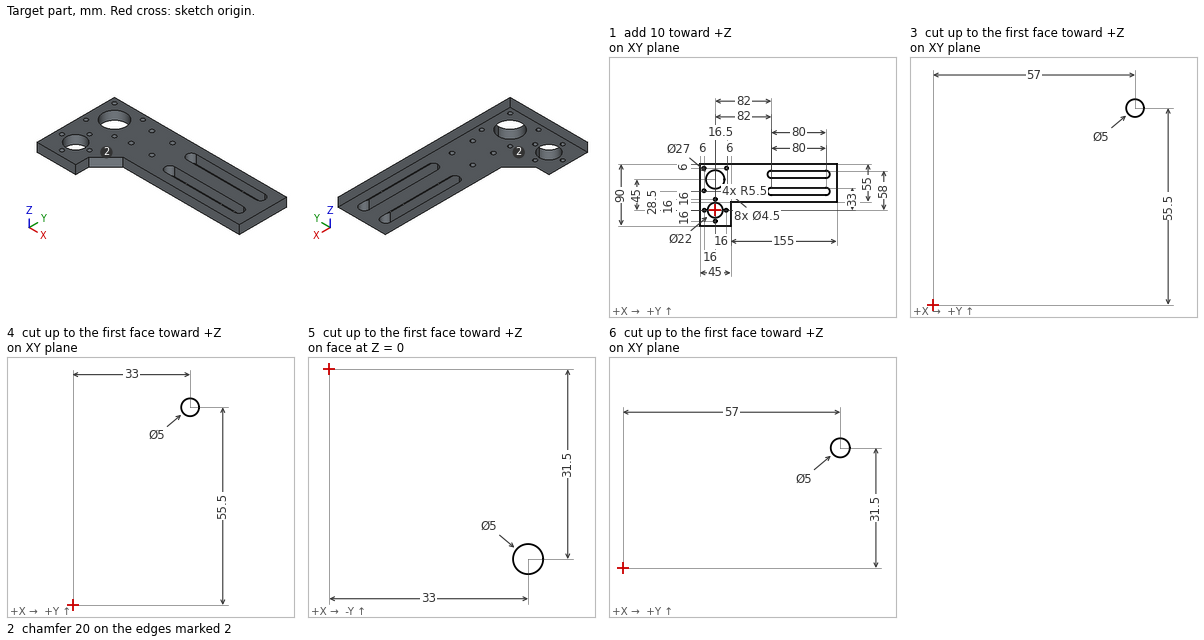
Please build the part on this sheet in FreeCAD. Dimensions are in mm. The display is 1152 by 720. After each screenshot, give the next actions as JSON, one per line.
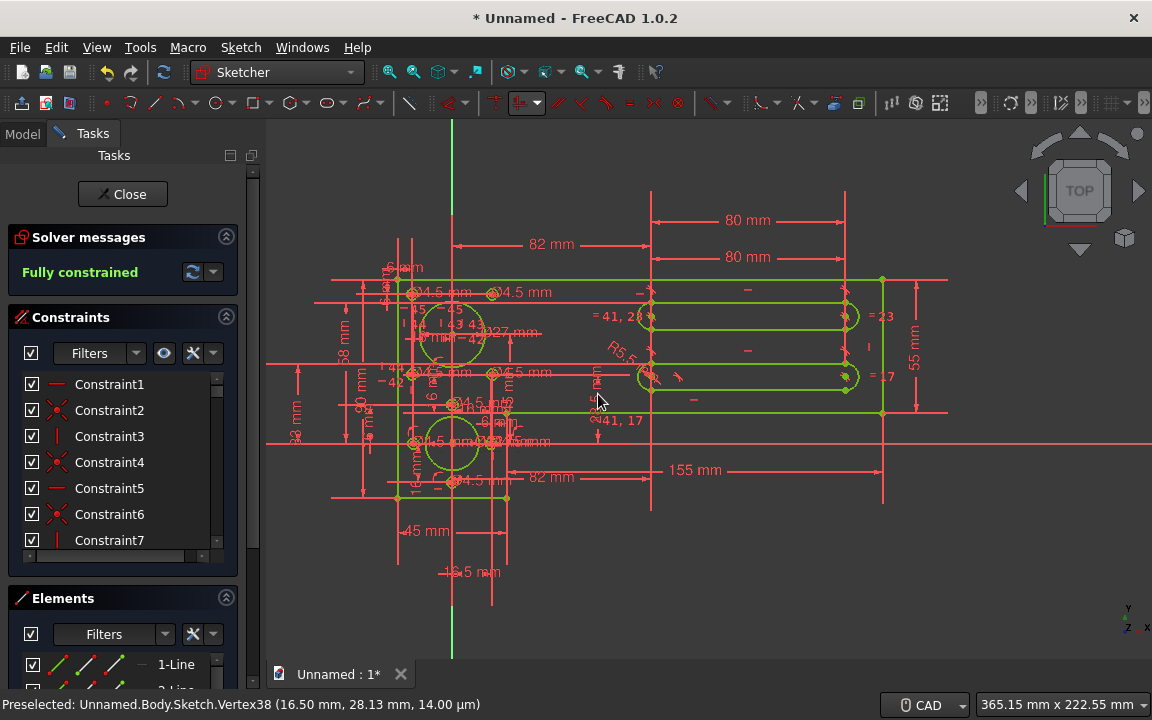
{"action": "left_click", "coordinate": [123, 194]}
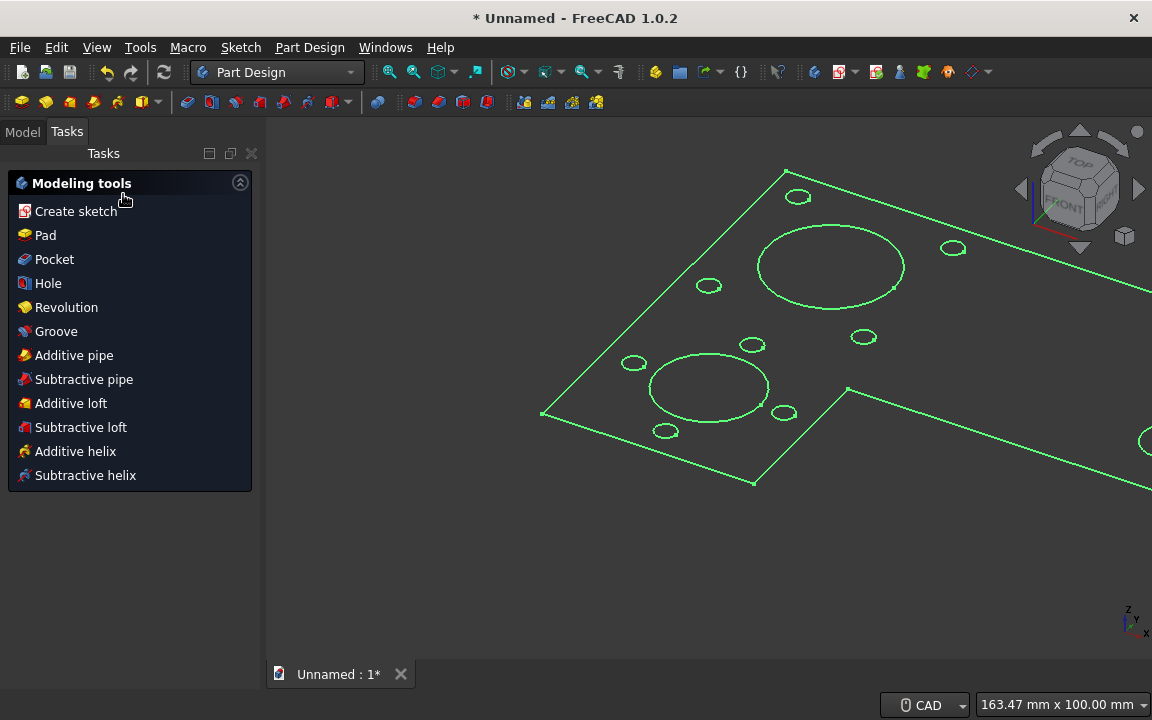
{"action": "left_click", "coordinate": [22, 102]}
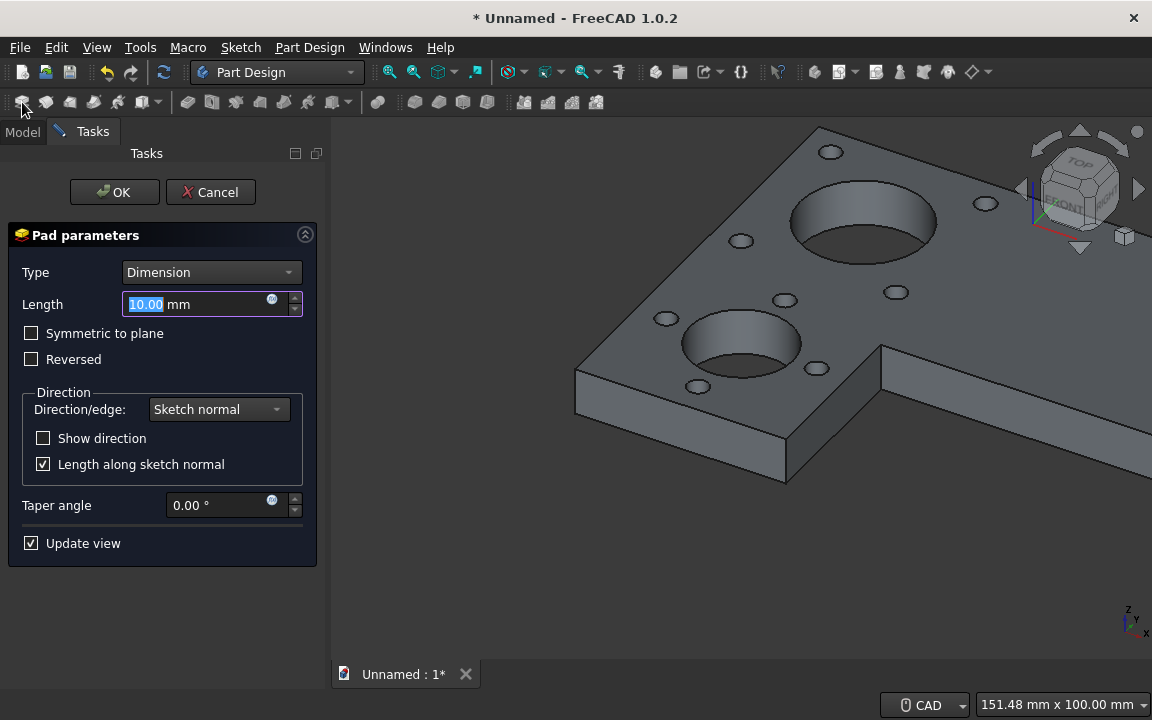
{"action": "type", "text": "10"}
{"action": "key", "text": "Tab"}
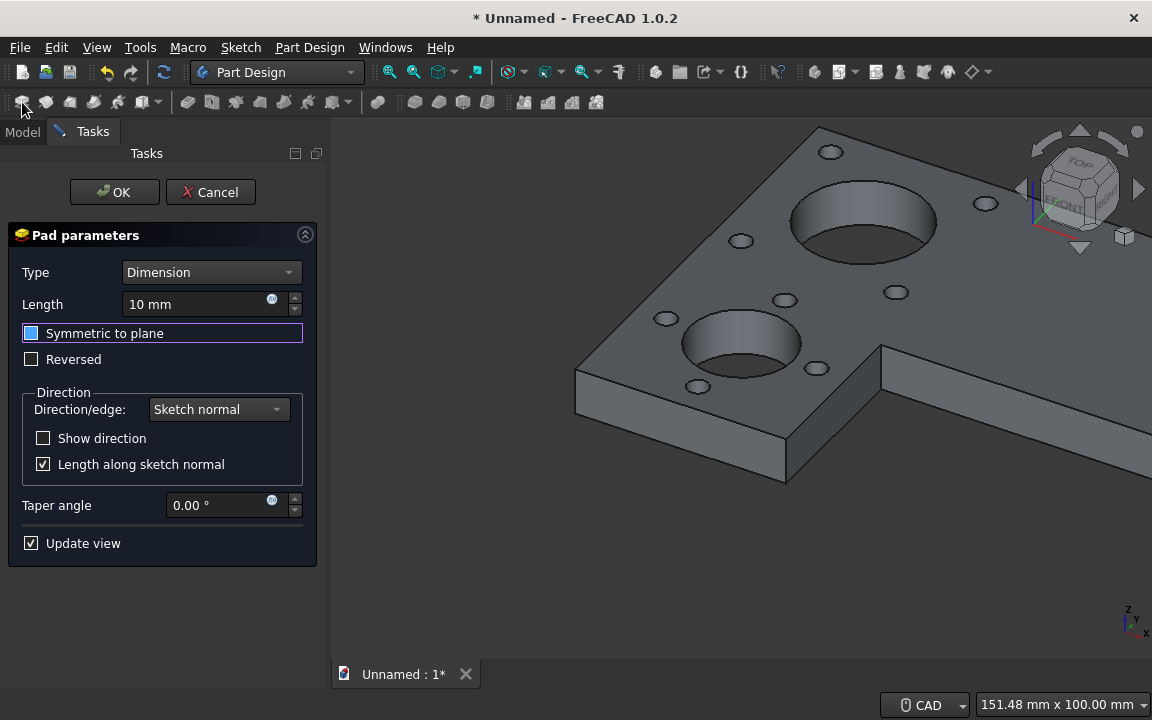
{"action": "left_click", "coordinate": [115, 192]}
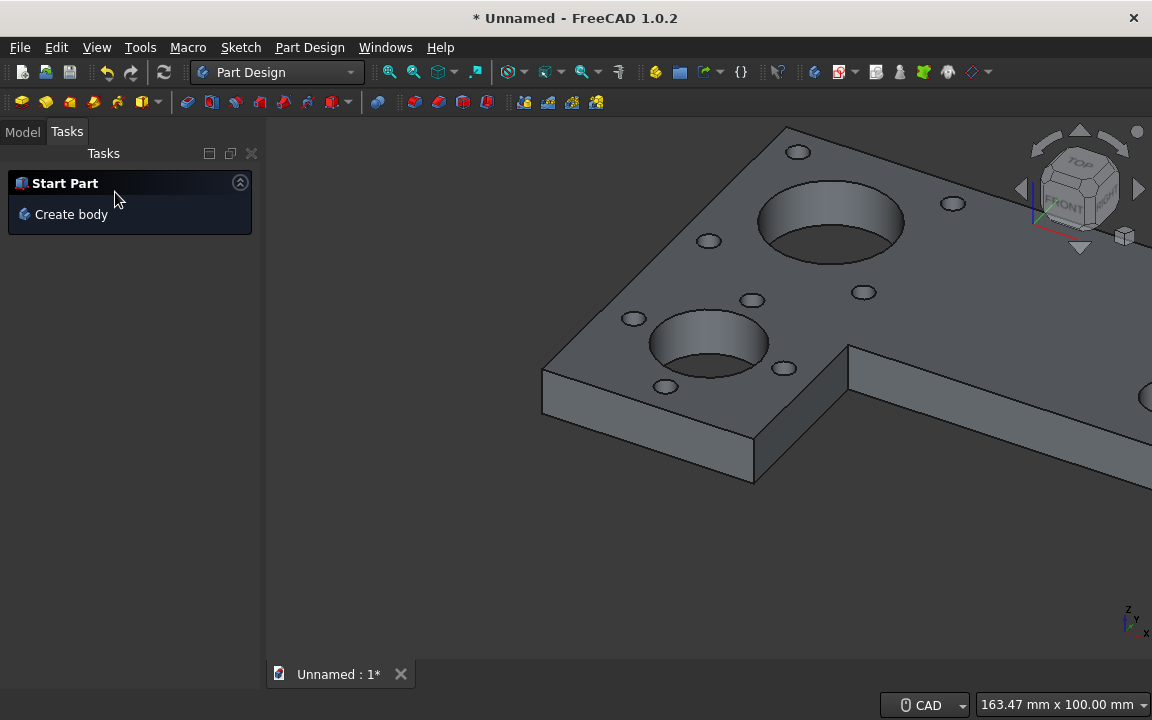
{"action": "key", "text": "v f"}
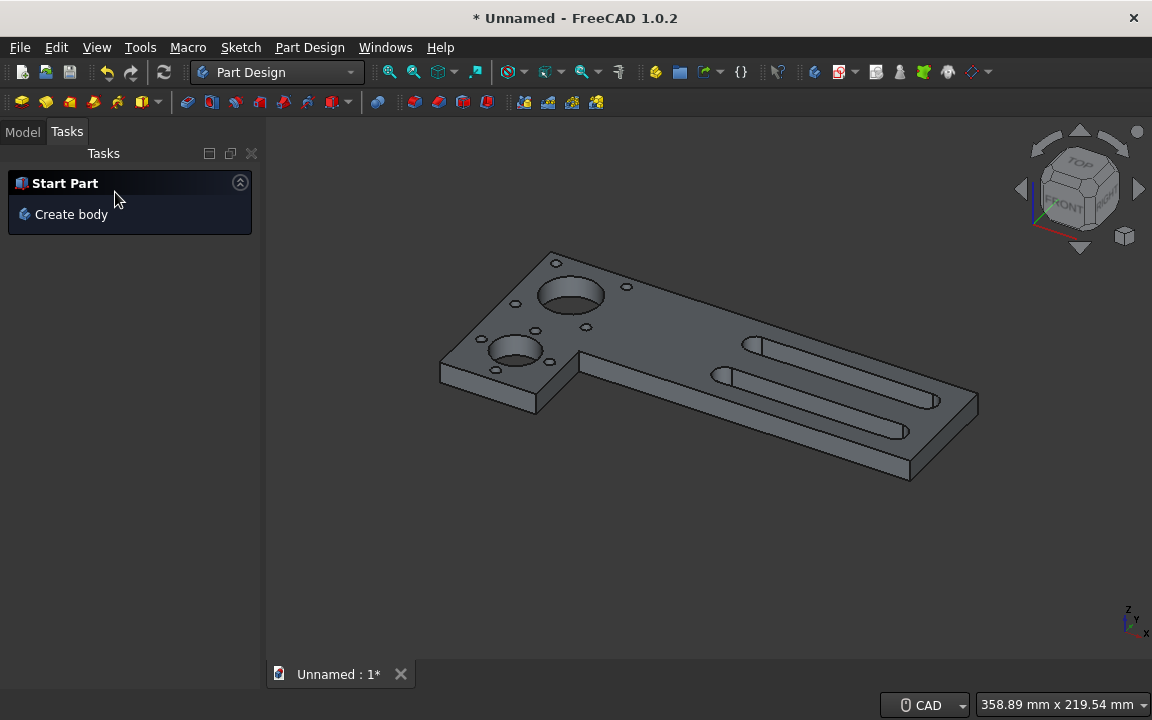
{"action": "key", "text": "0"}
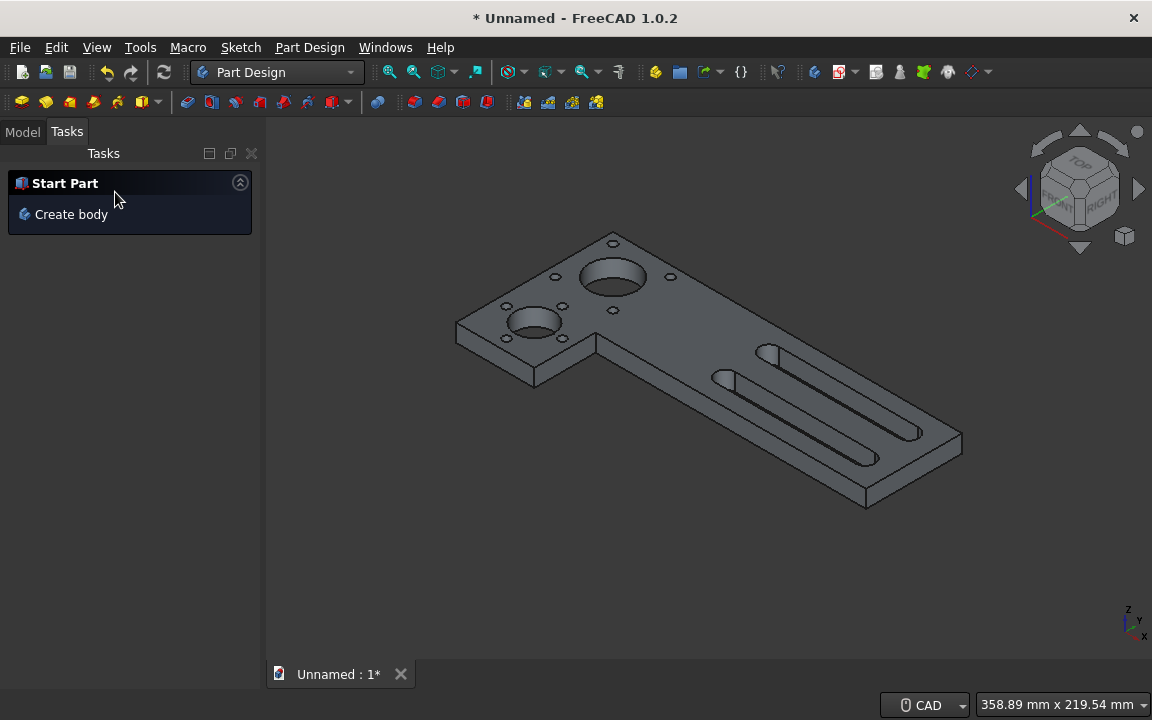
{"action": "key", "text": "2"}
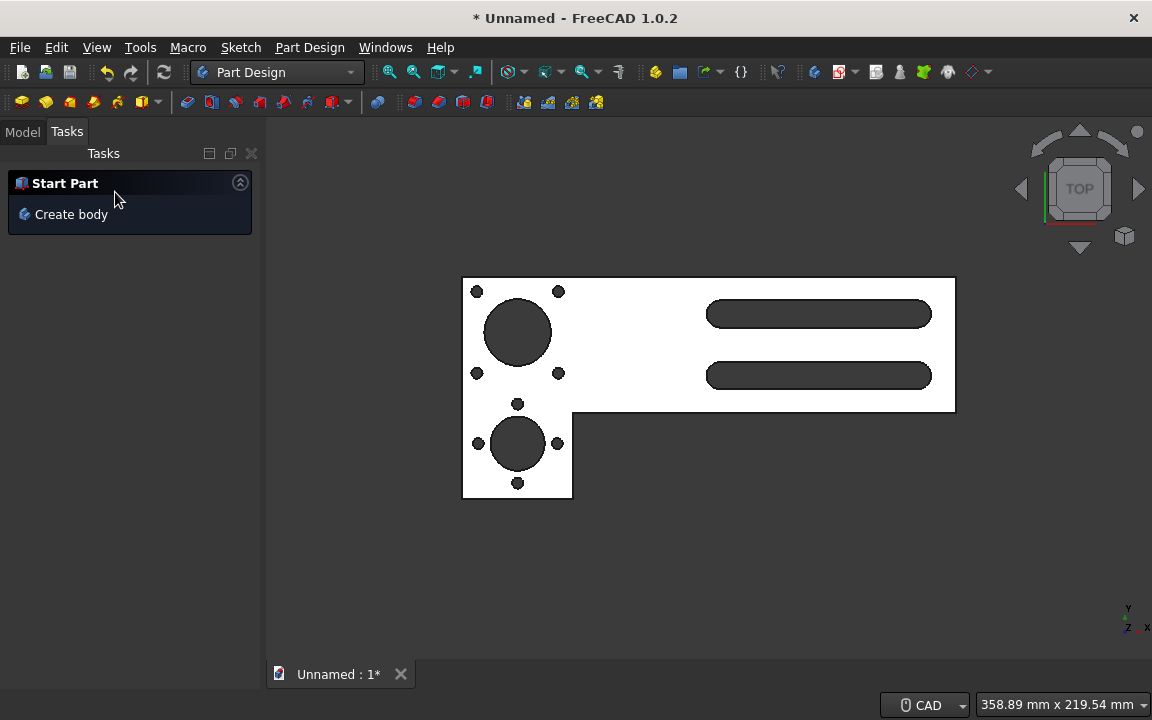
{"action": "key", "text": "1"}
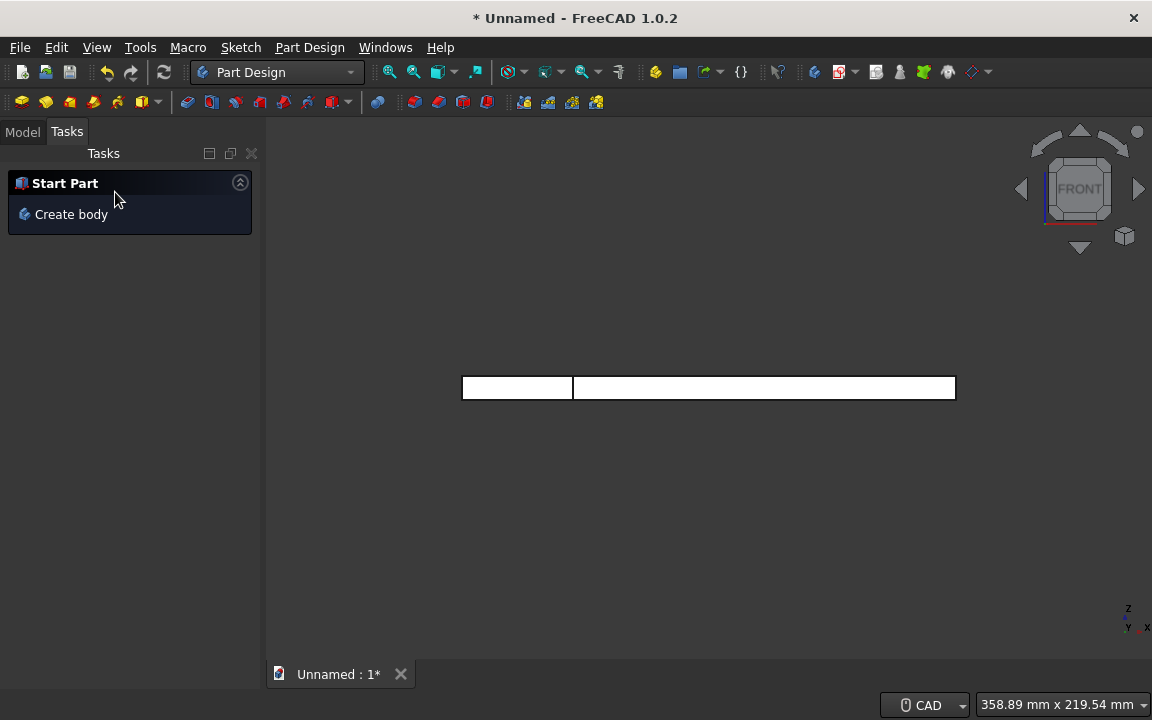
{"action": "key", "text": "3"}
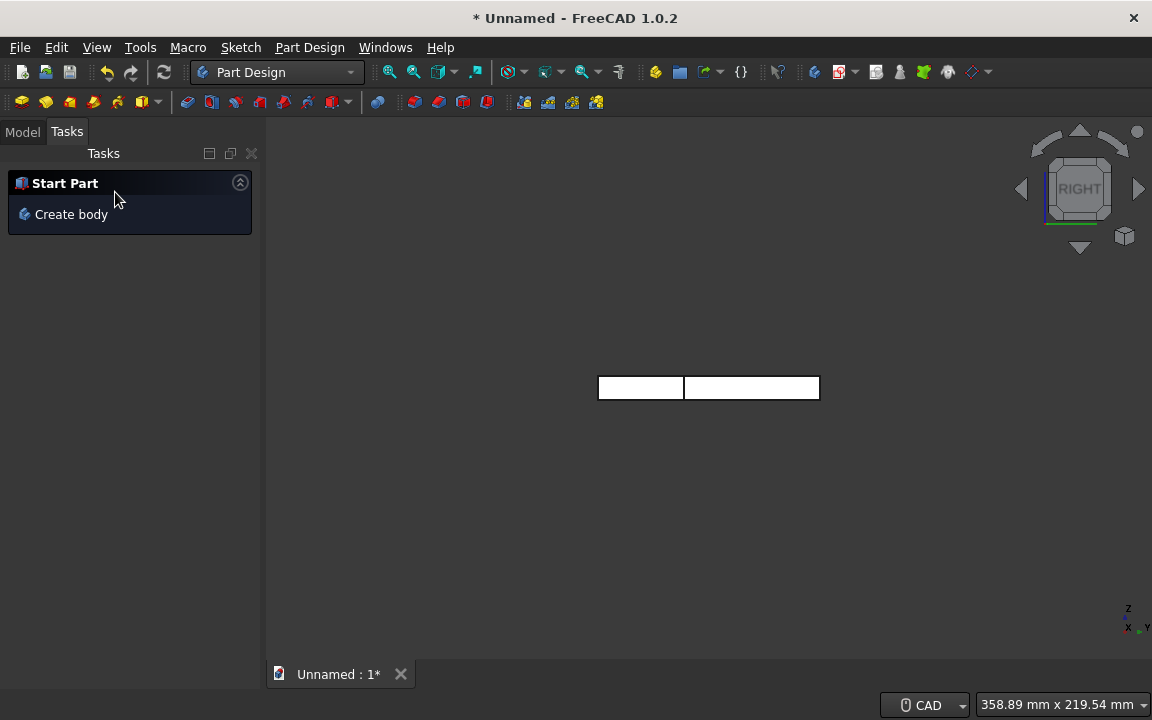
{"action": "key", "text": "v f"}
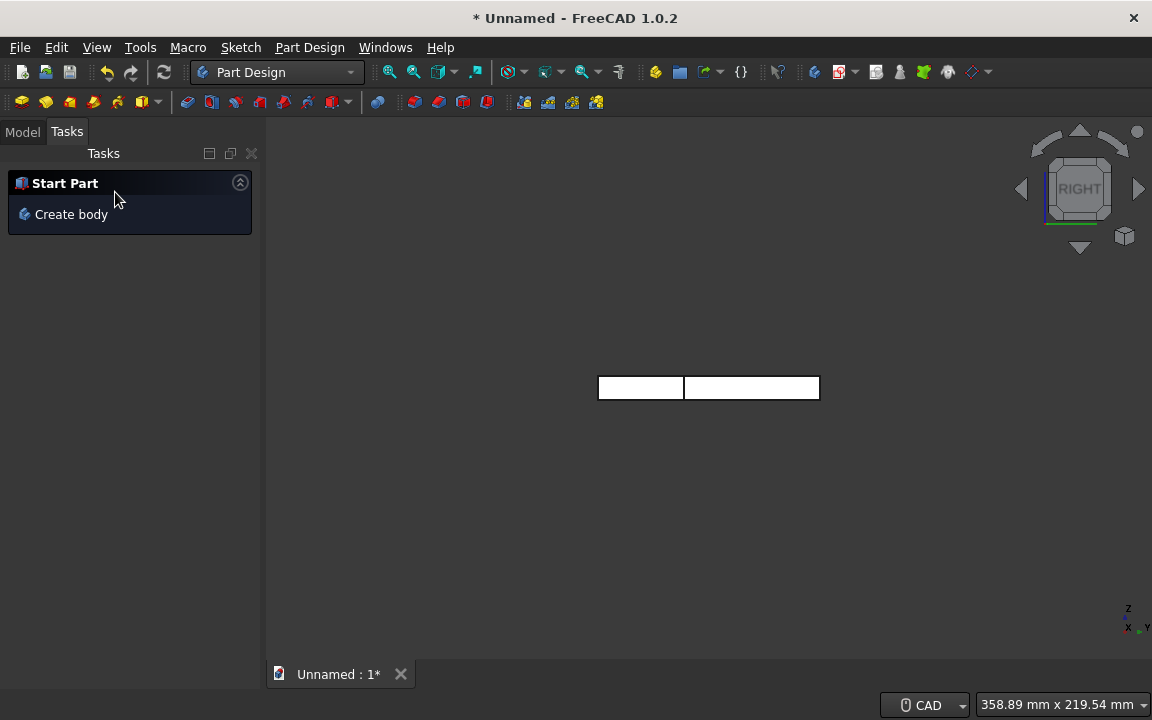
{"action": "key", "text": "5"}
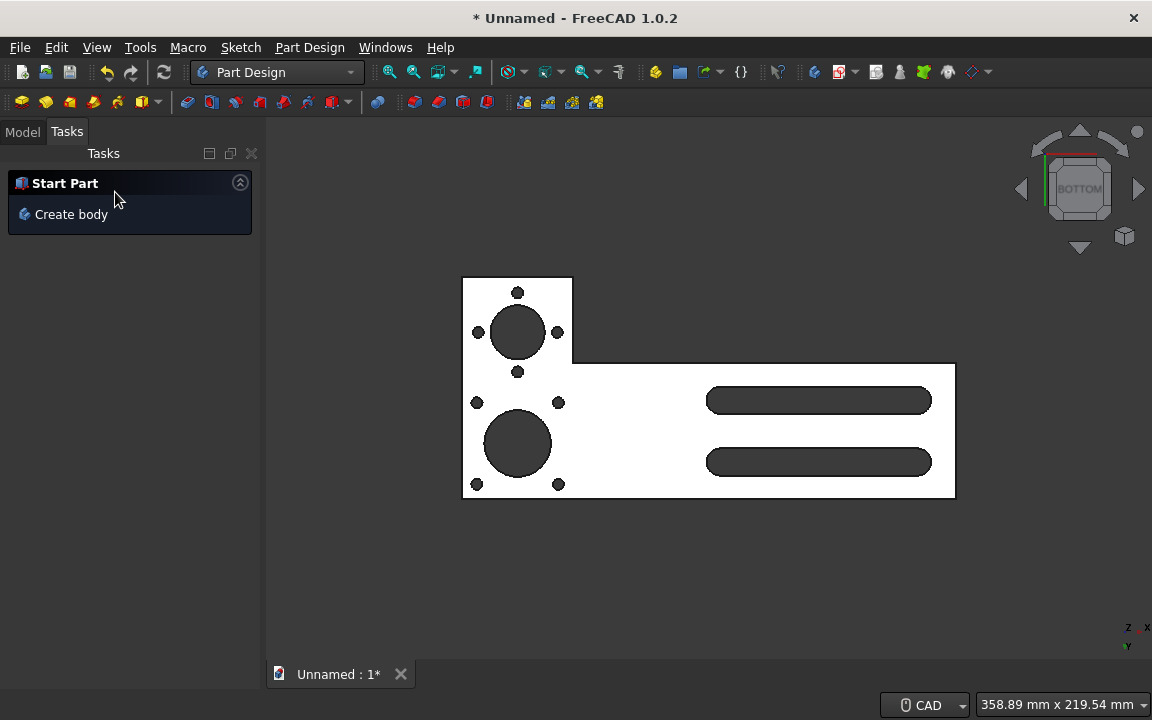
{"action": "key", "text": "4"}